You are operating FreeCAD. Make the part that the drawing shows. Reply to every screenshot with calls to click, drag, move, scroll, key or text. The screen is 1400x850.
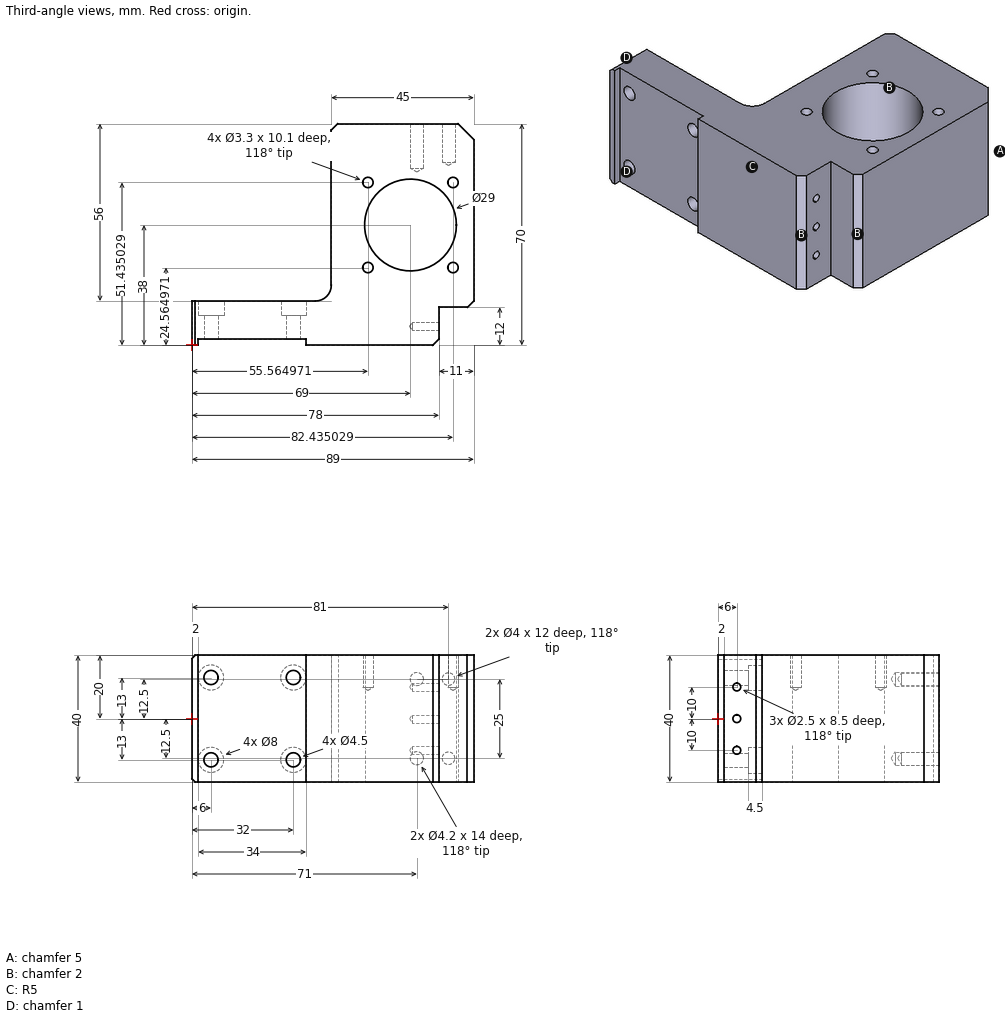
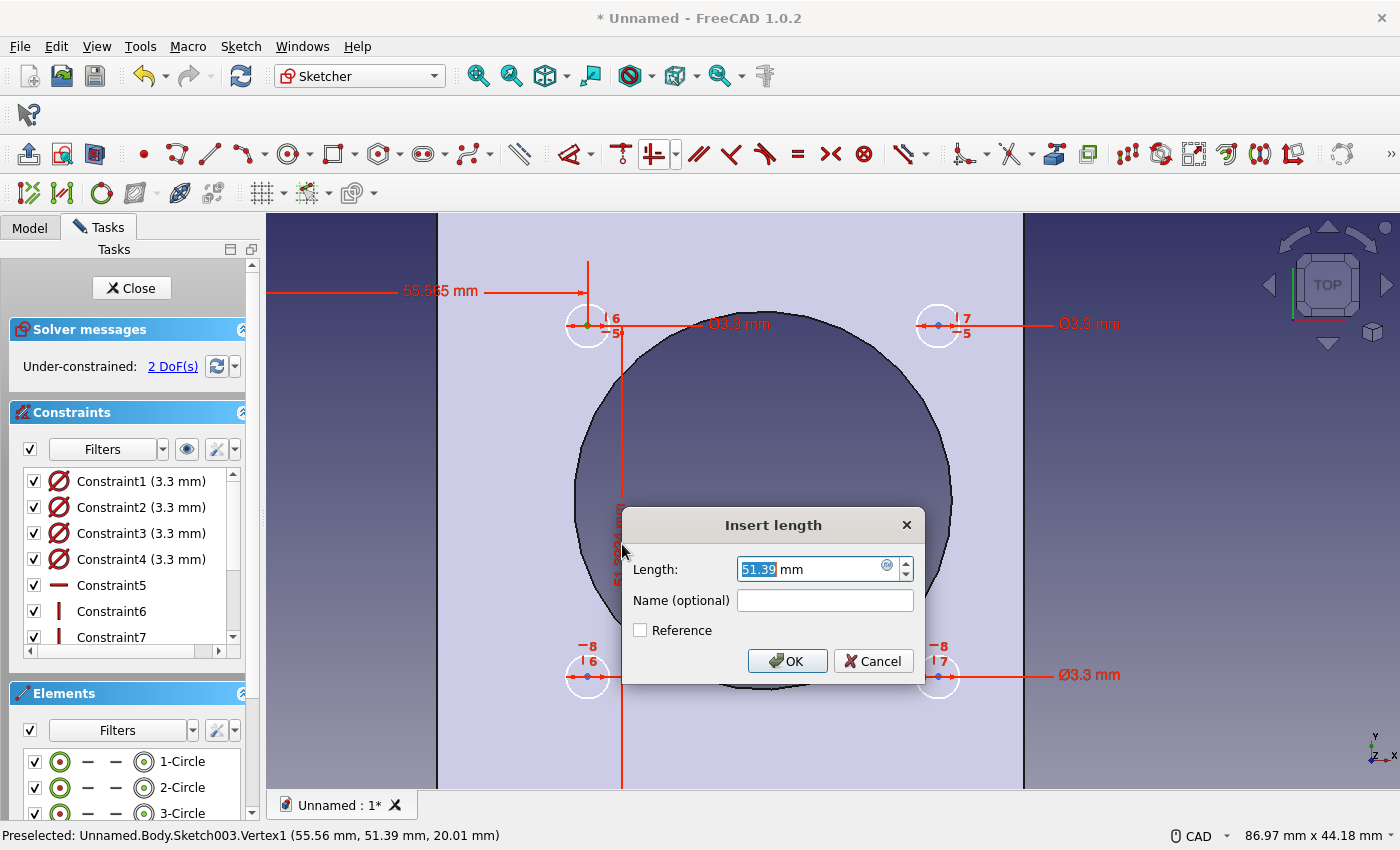
text(51.435029)
key(Return)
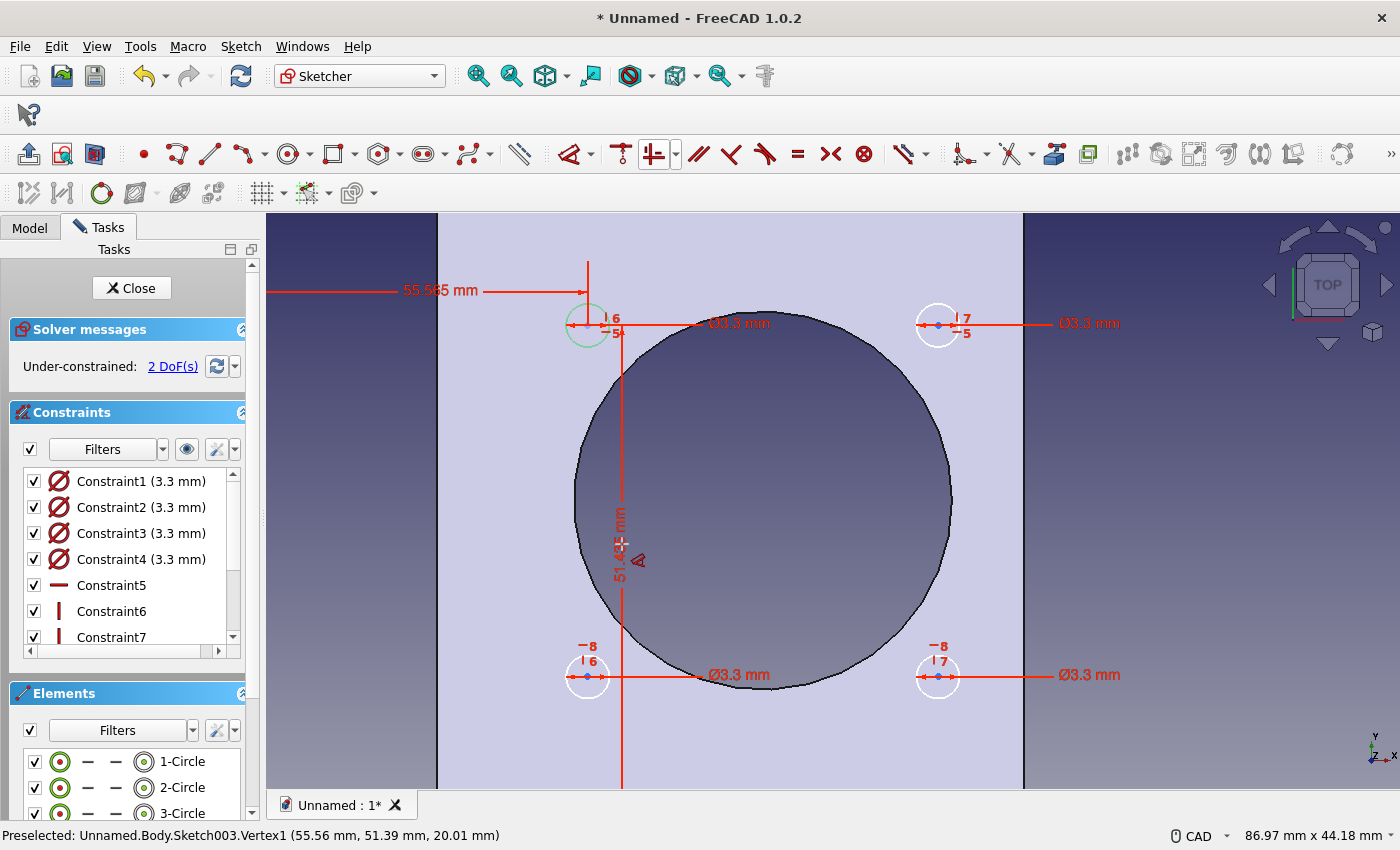
click(938, 325)
click(616, 291)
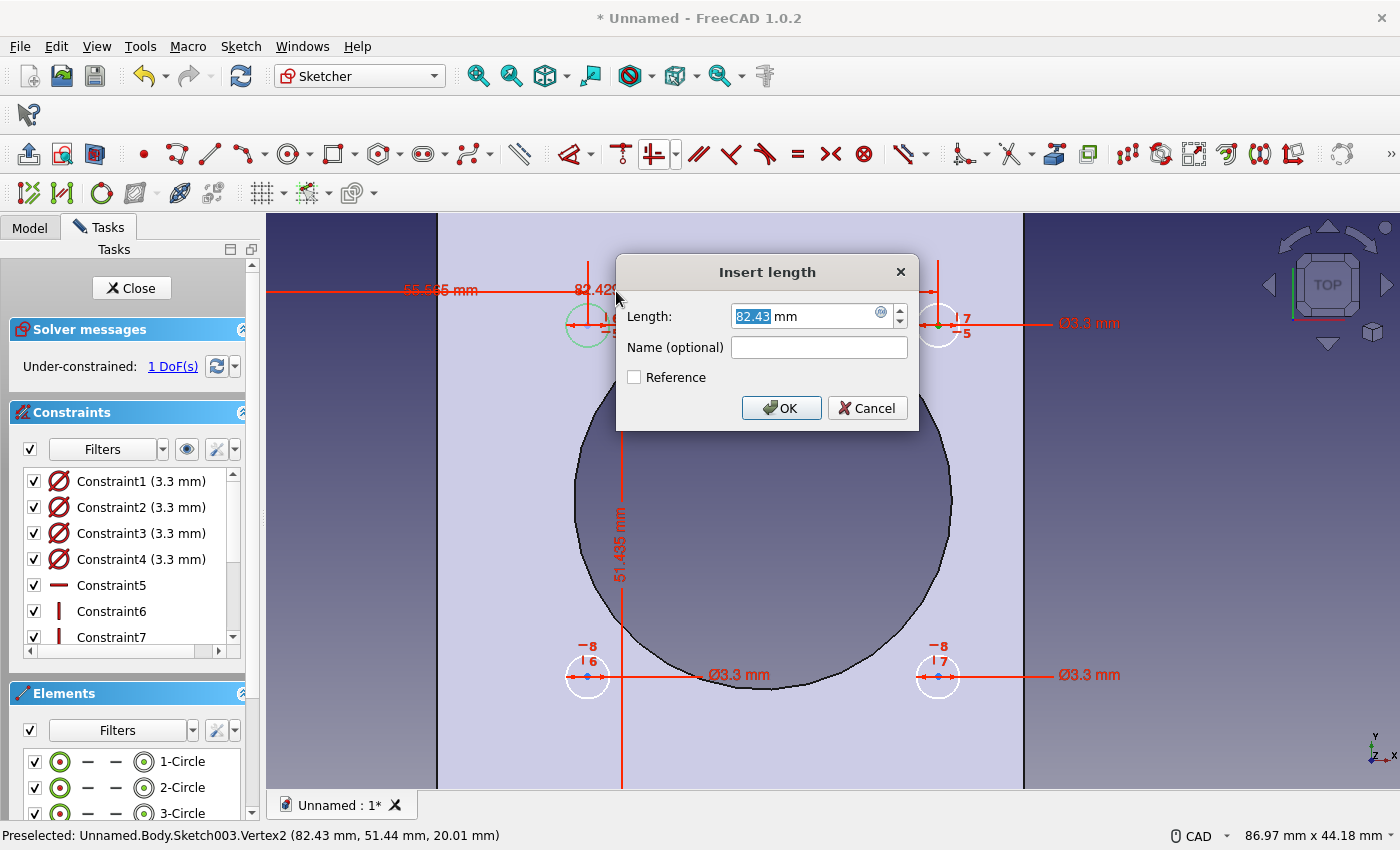
text(82.435029)
key(Return)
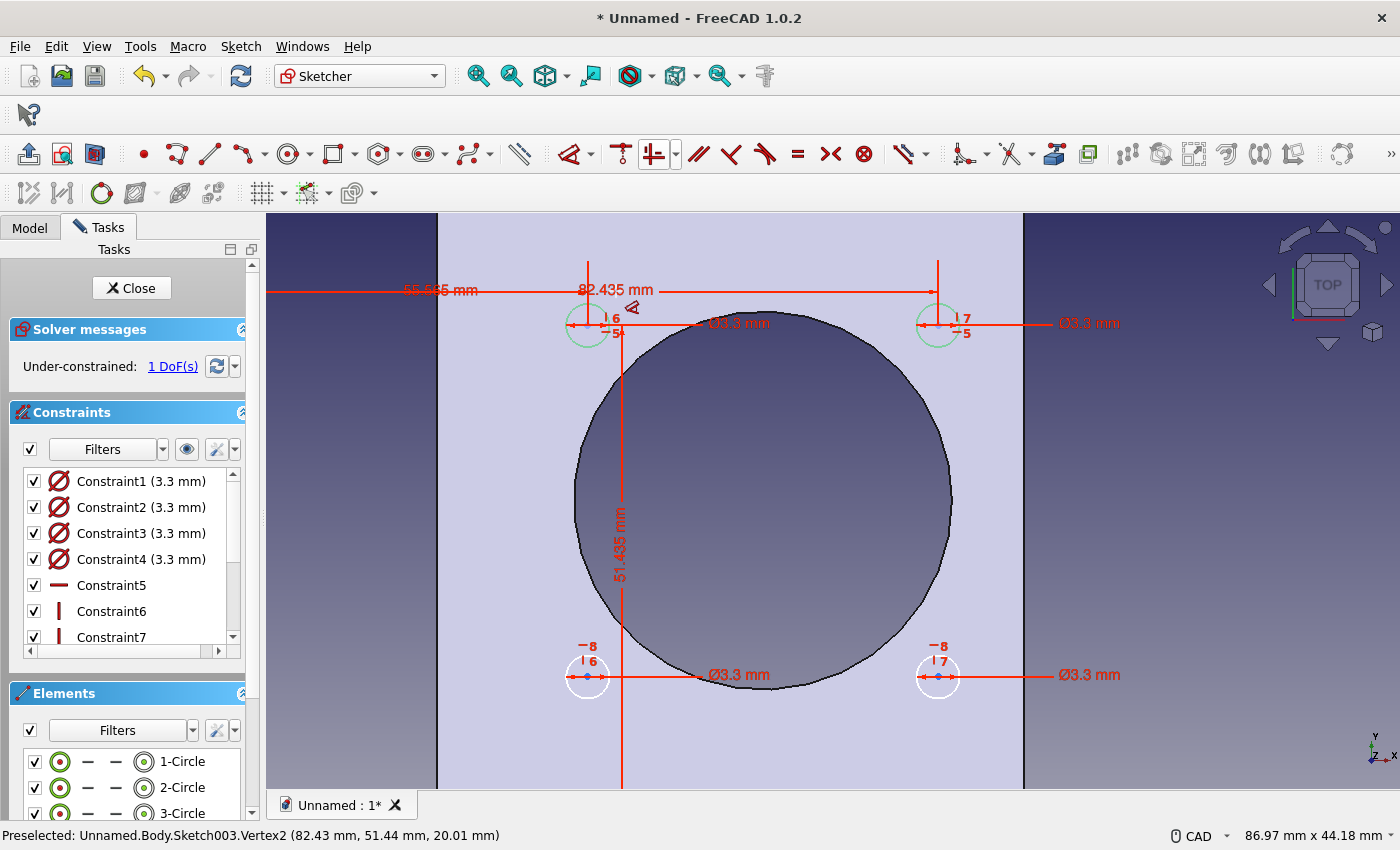
click(588, 677)
click(622, 719)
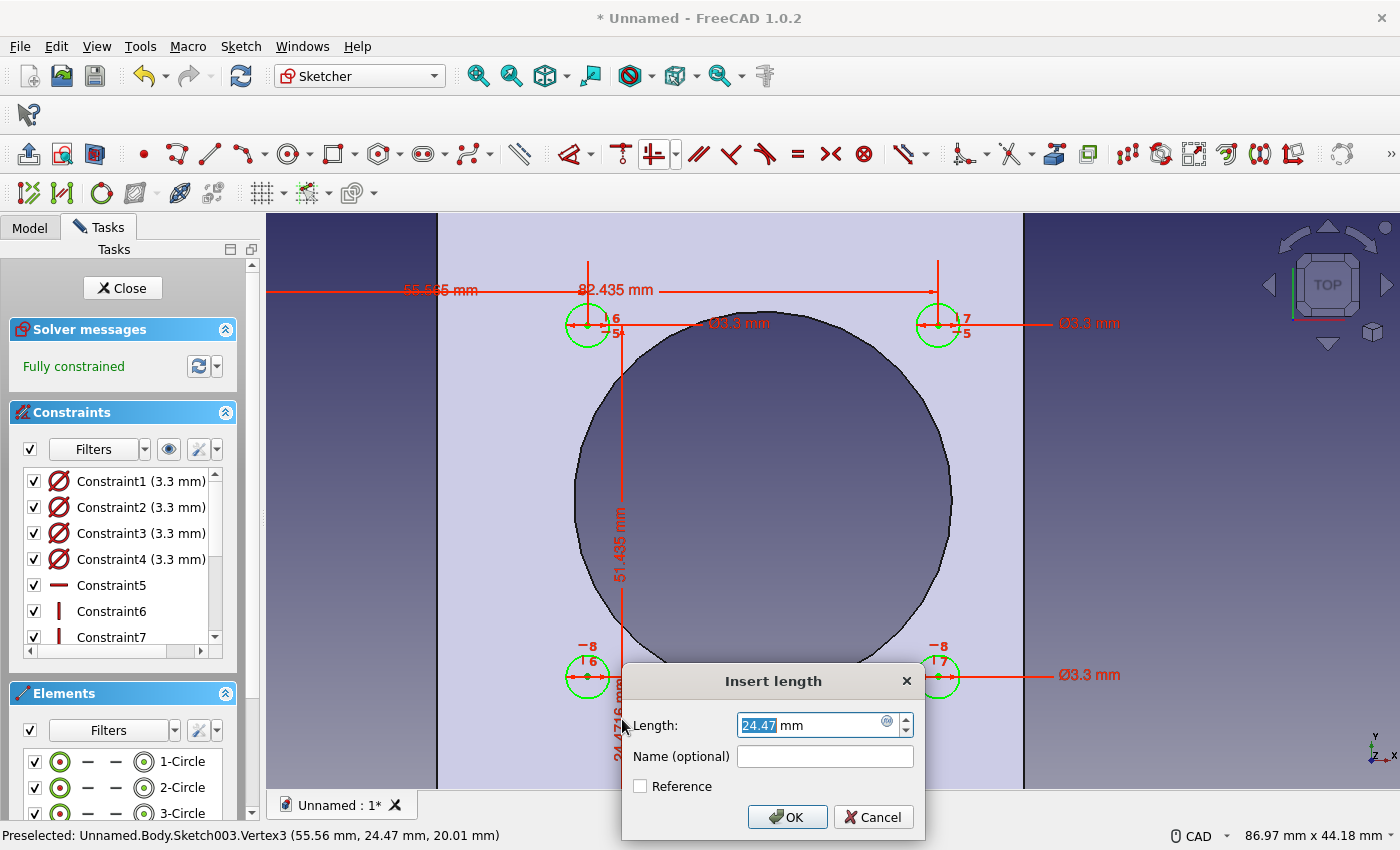
text(24.564971)
key(Return)
key(Escape)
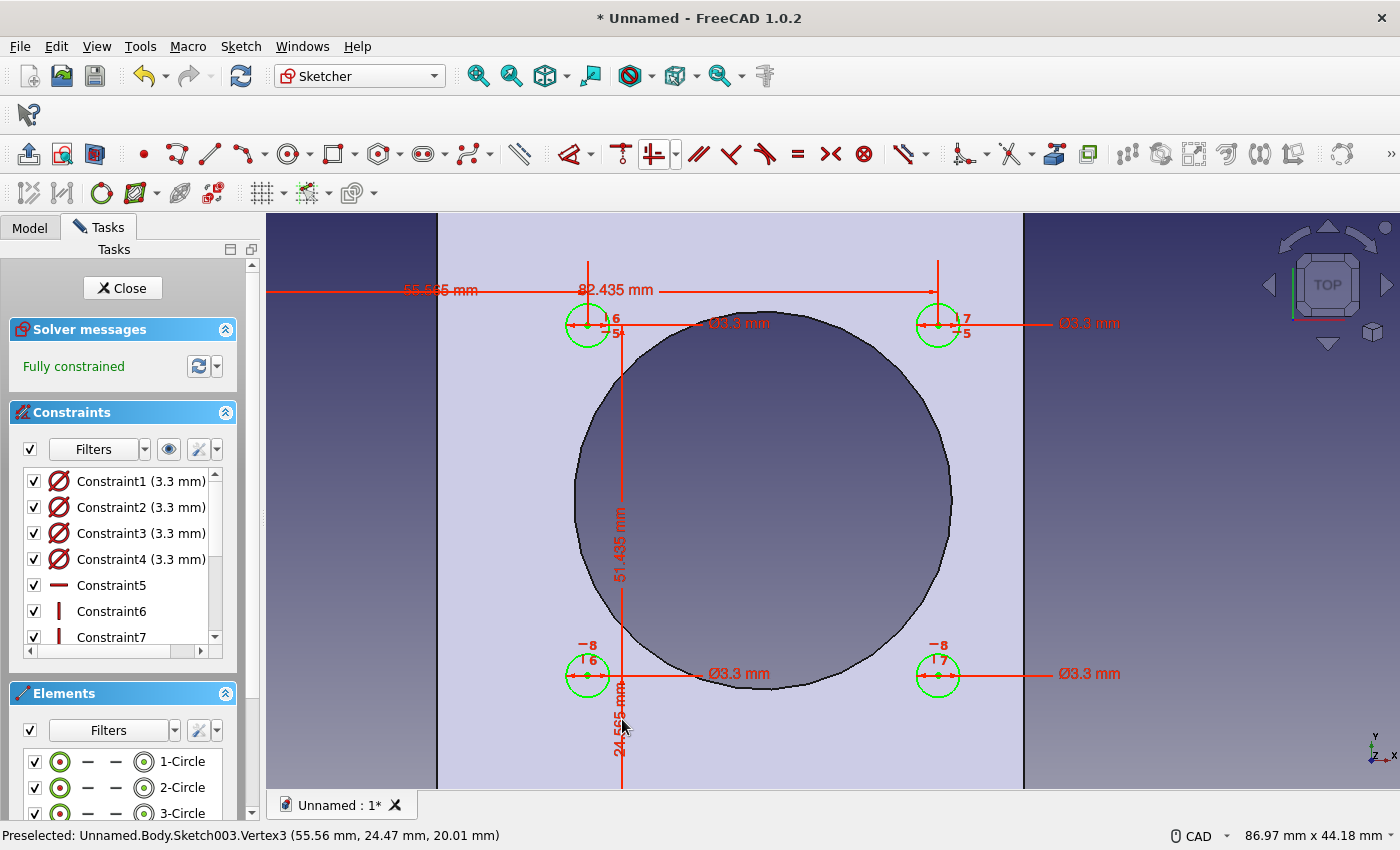
click(123, 288)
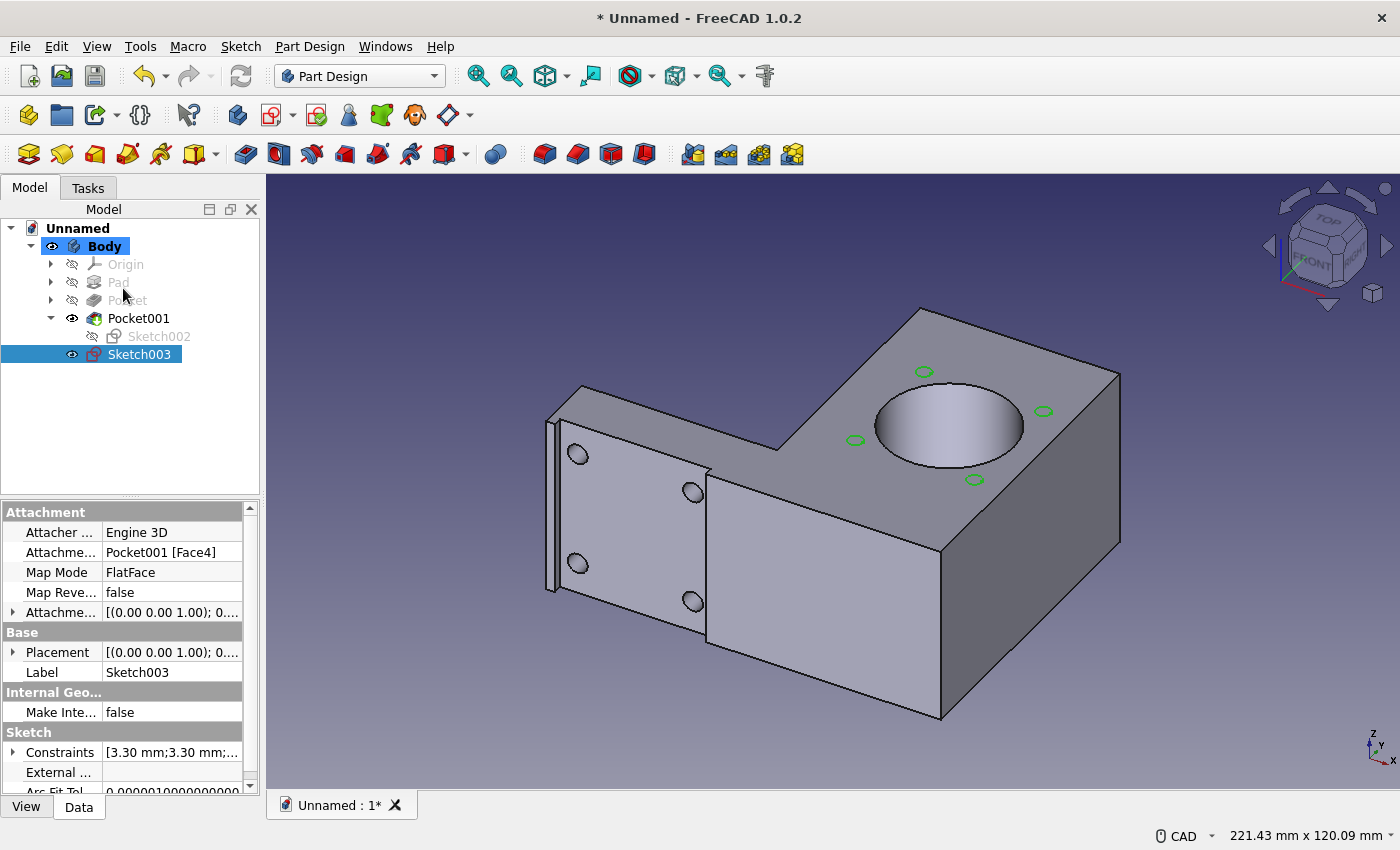
click(279, 154)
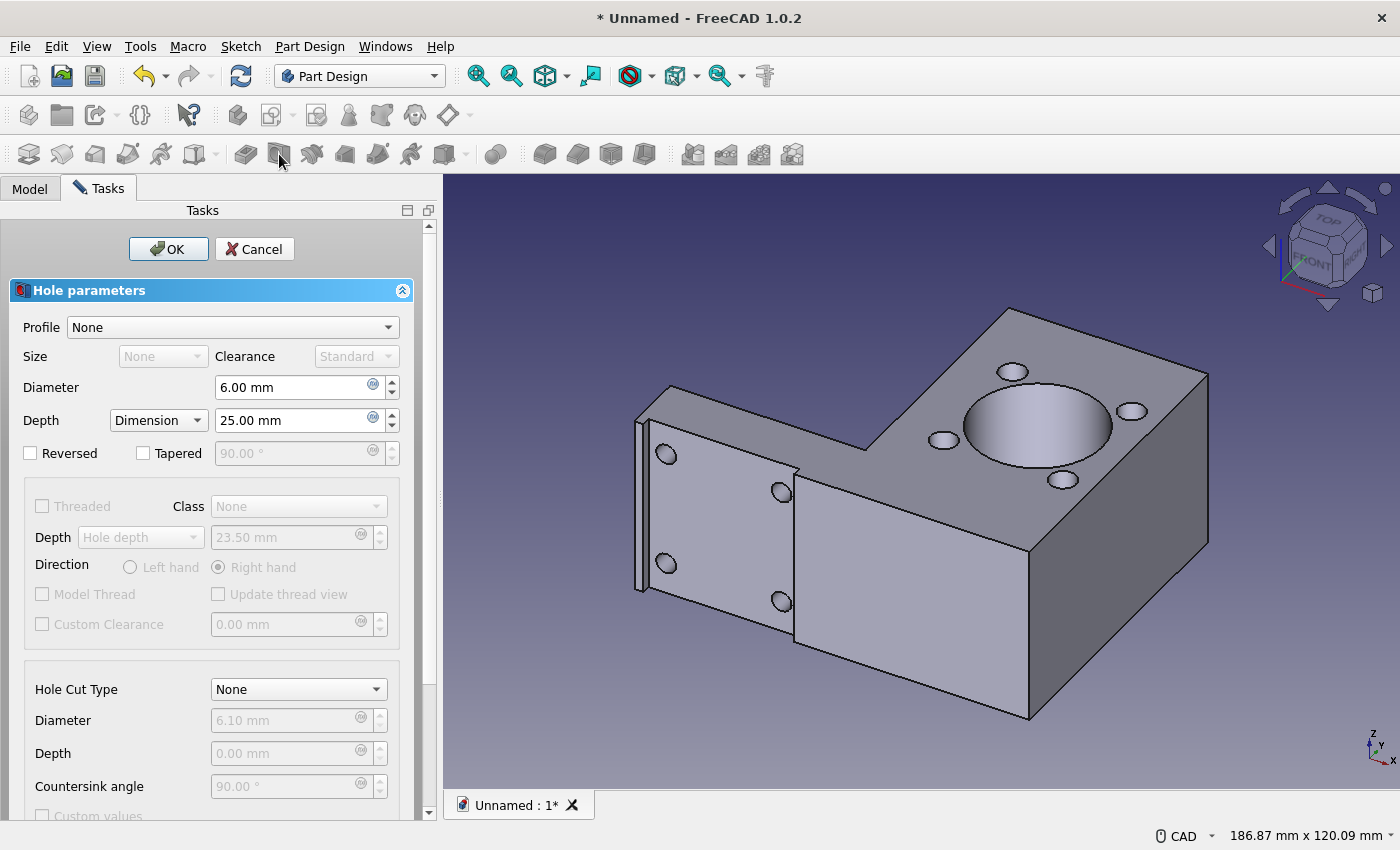
triple_click(300, 388)